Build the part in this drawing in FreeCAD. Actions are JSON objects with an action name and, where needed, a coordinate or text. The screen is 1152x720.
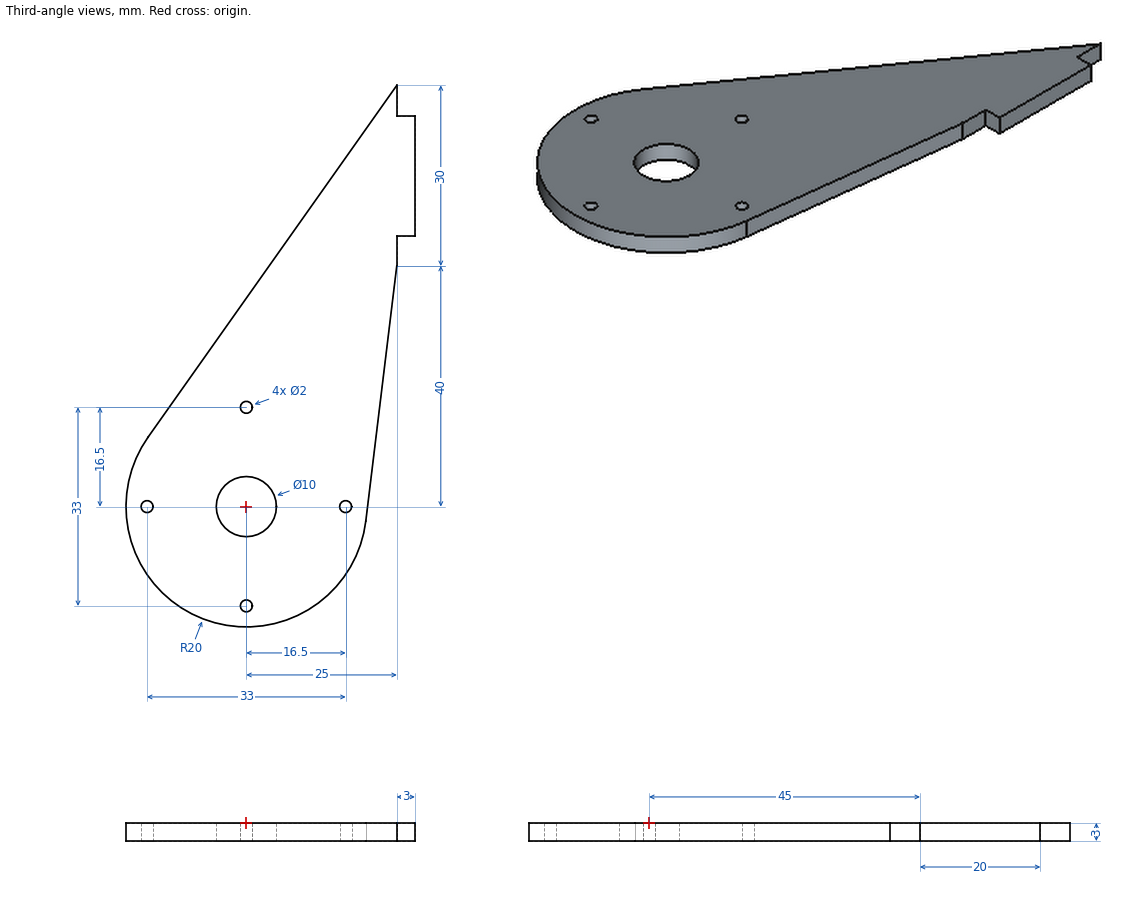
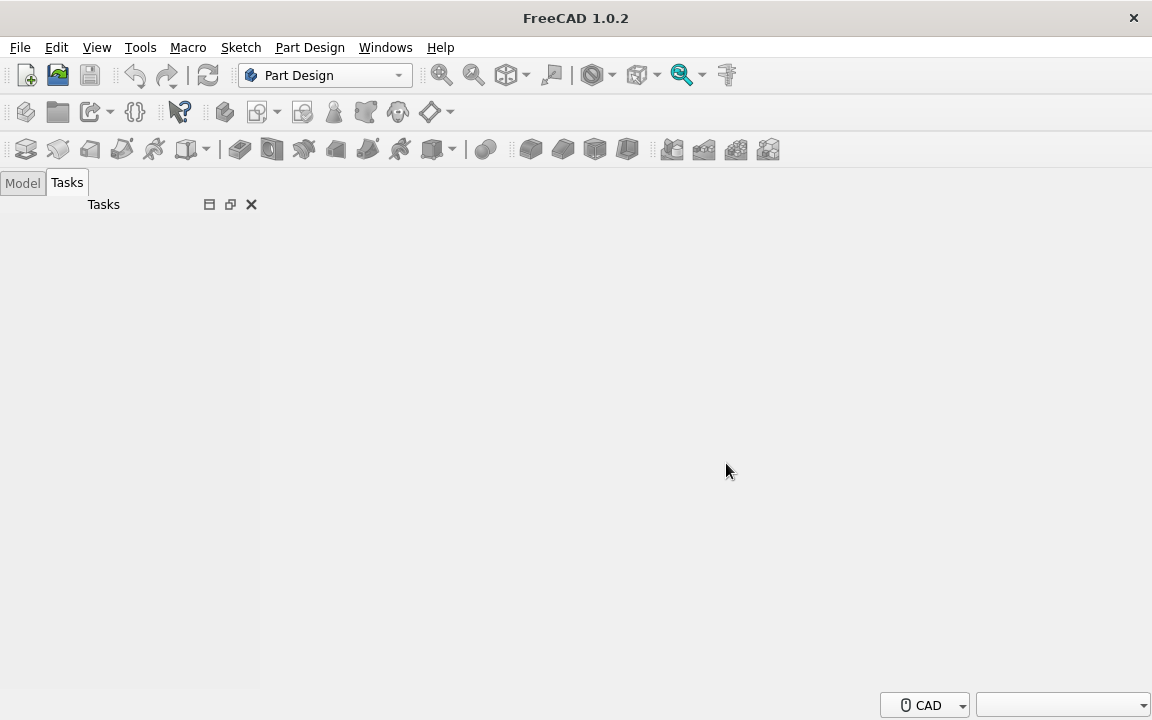
{"action": "left_click", "coordinate": [26, 76]}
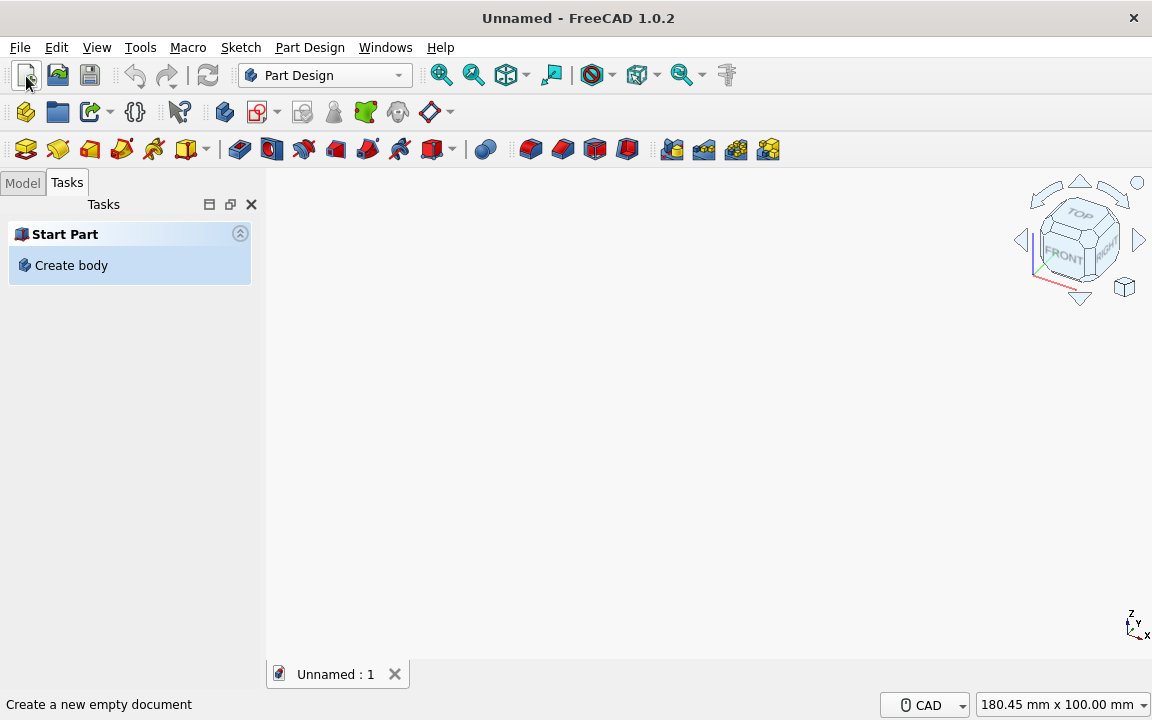
{"action": "left_click", "coordinate": [258, 112]}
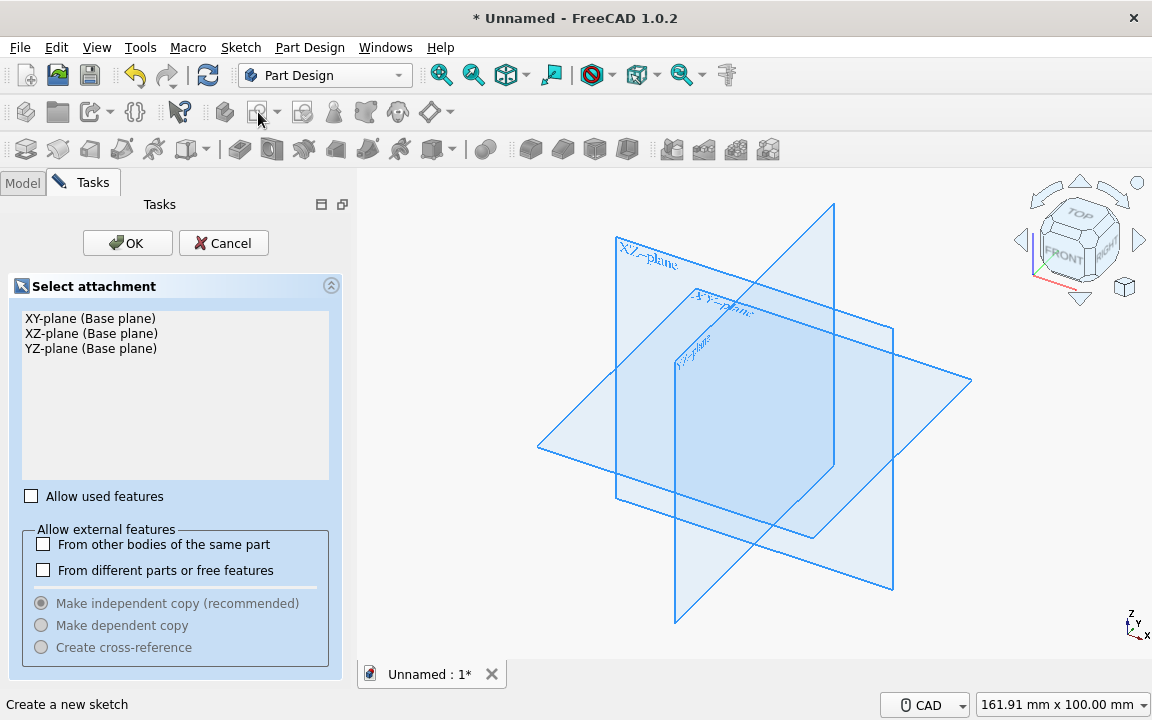
{"action": "left_click", "coordinate": [82, 318]}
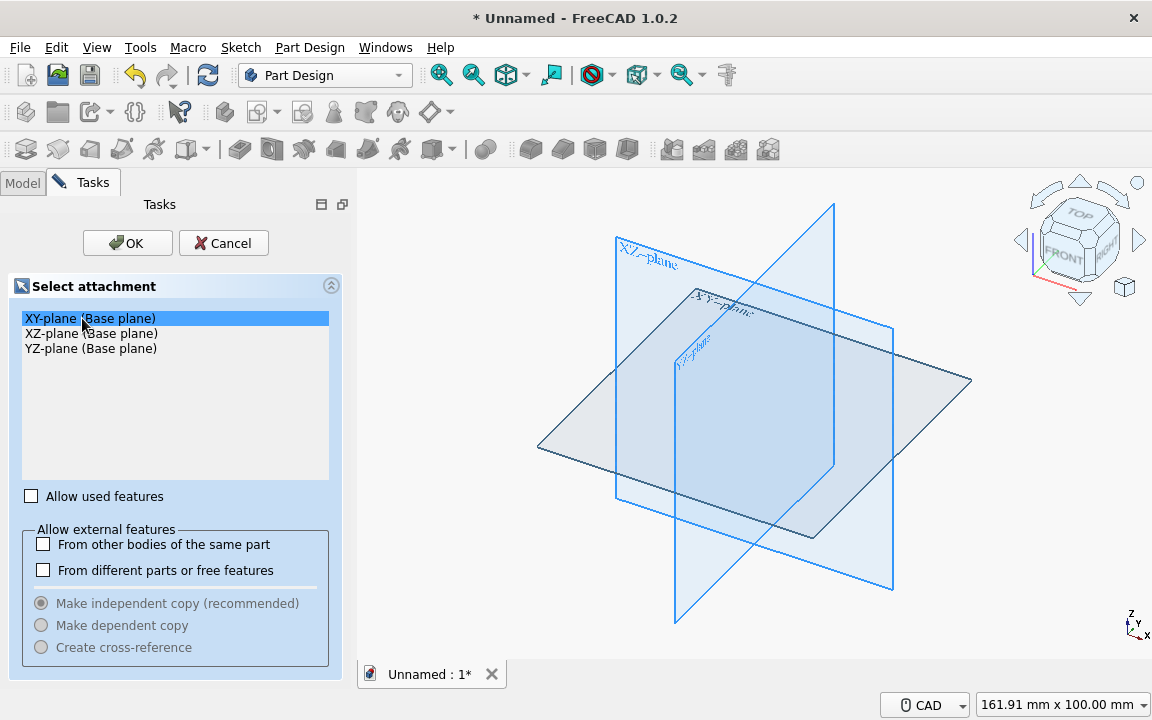
{"action": "left_click", "coordinate": [128, 243]}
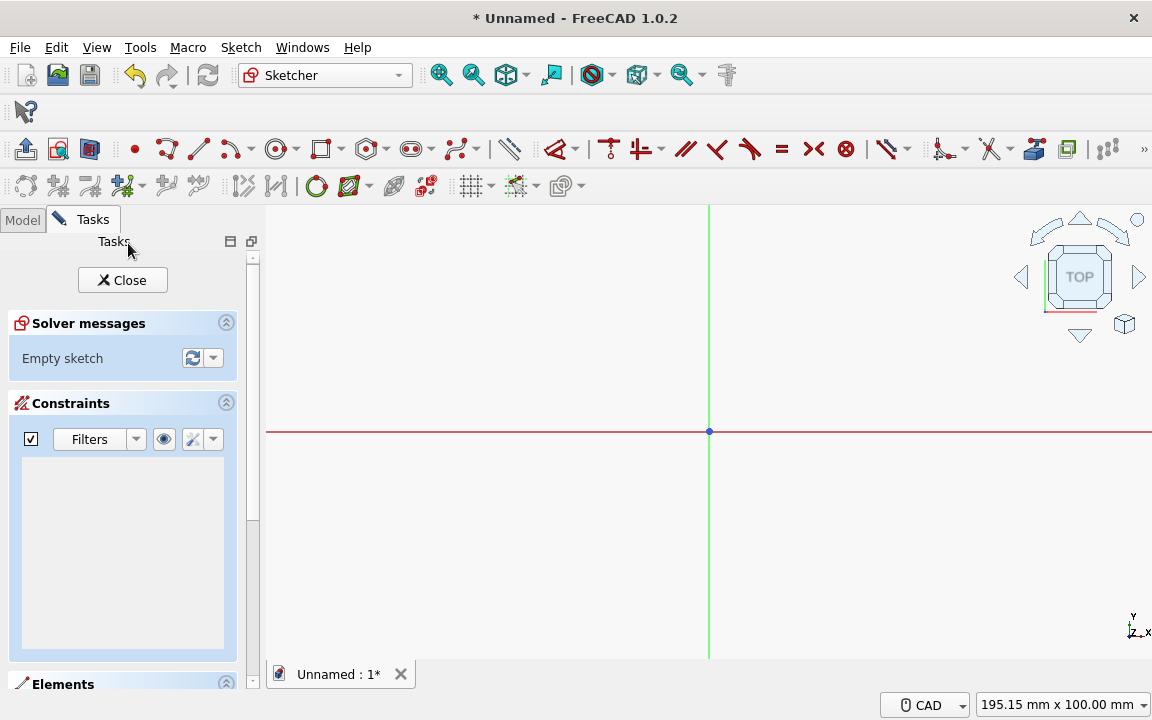
{"action": "scroll", "coordinate": [461, 631], "scroll_direction": "down", "scroll_amount": 2}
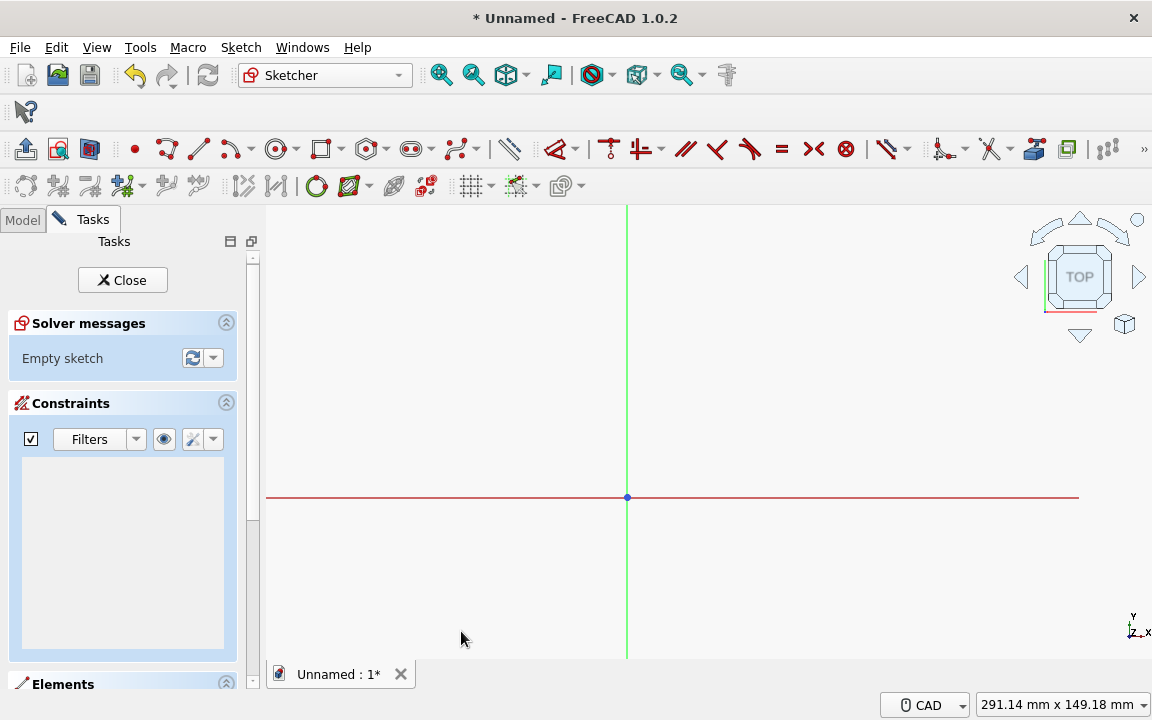
{"action": "left_click", "coordinate": [168, 150]}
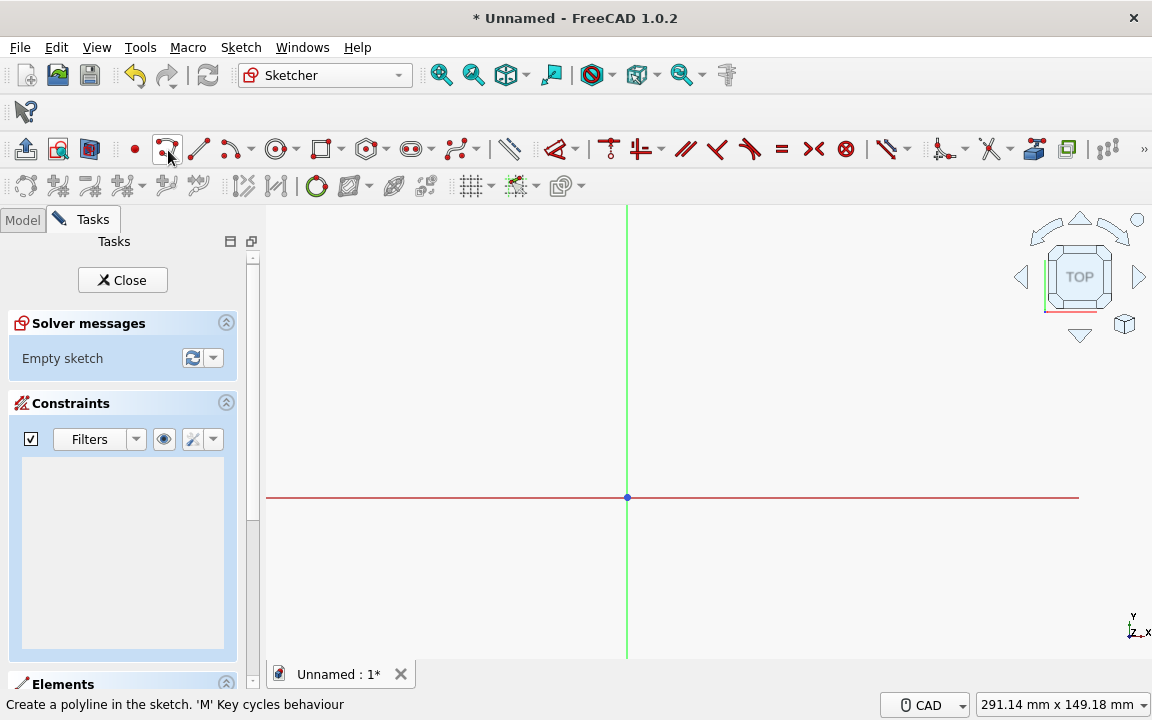
{"action": "scroll", "coordinate": [688, 505], "scroll_direction": "up", "scroll_amount": 4}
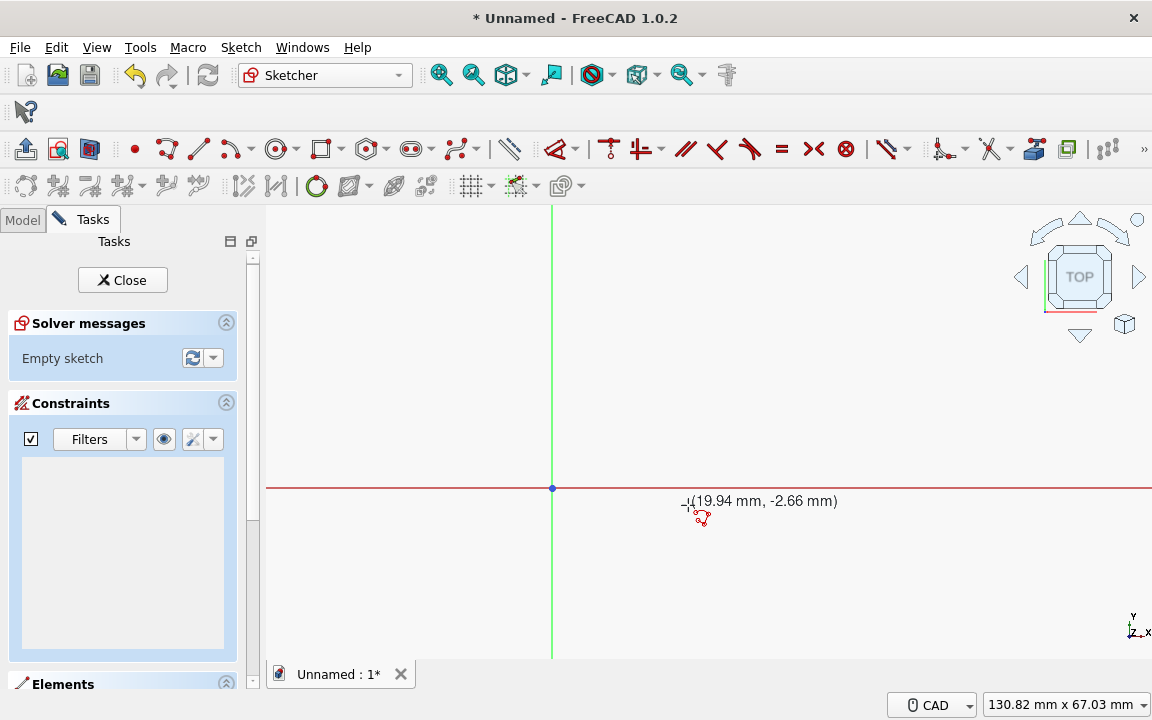
{"action": "left_click", "coordinate": [687, 505]}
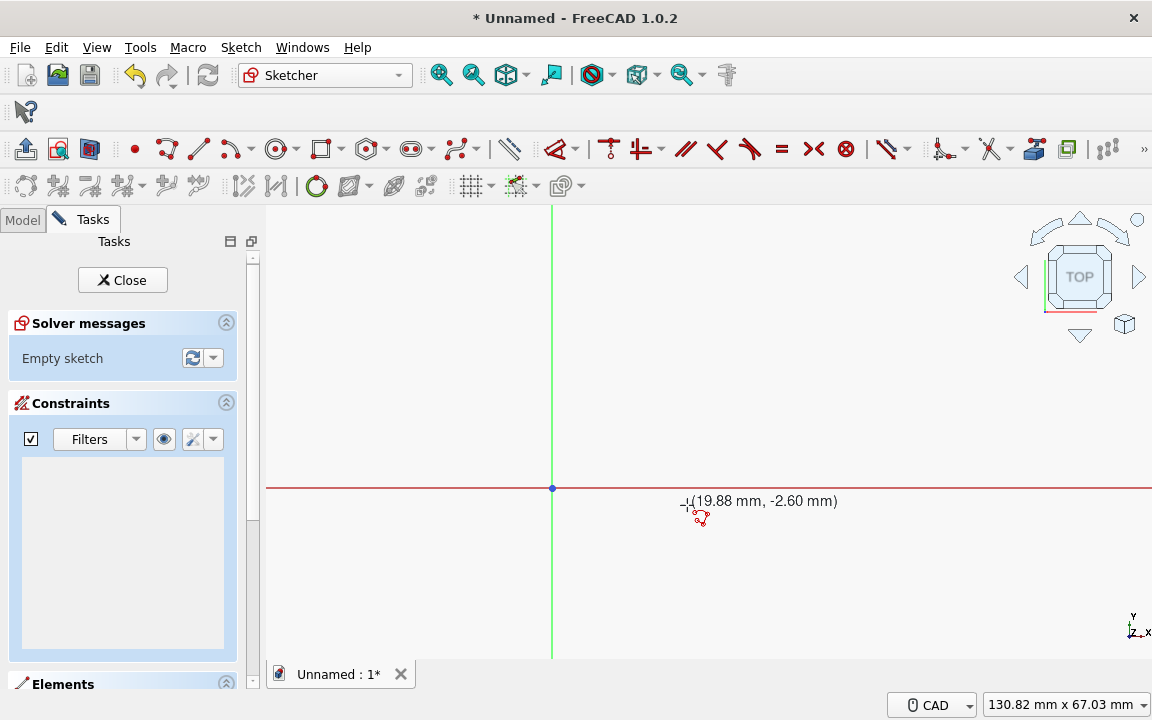
{"action": "scroll", "coordinate": [688, 528], "scroll_direction": "down", "scroll_amount": 4}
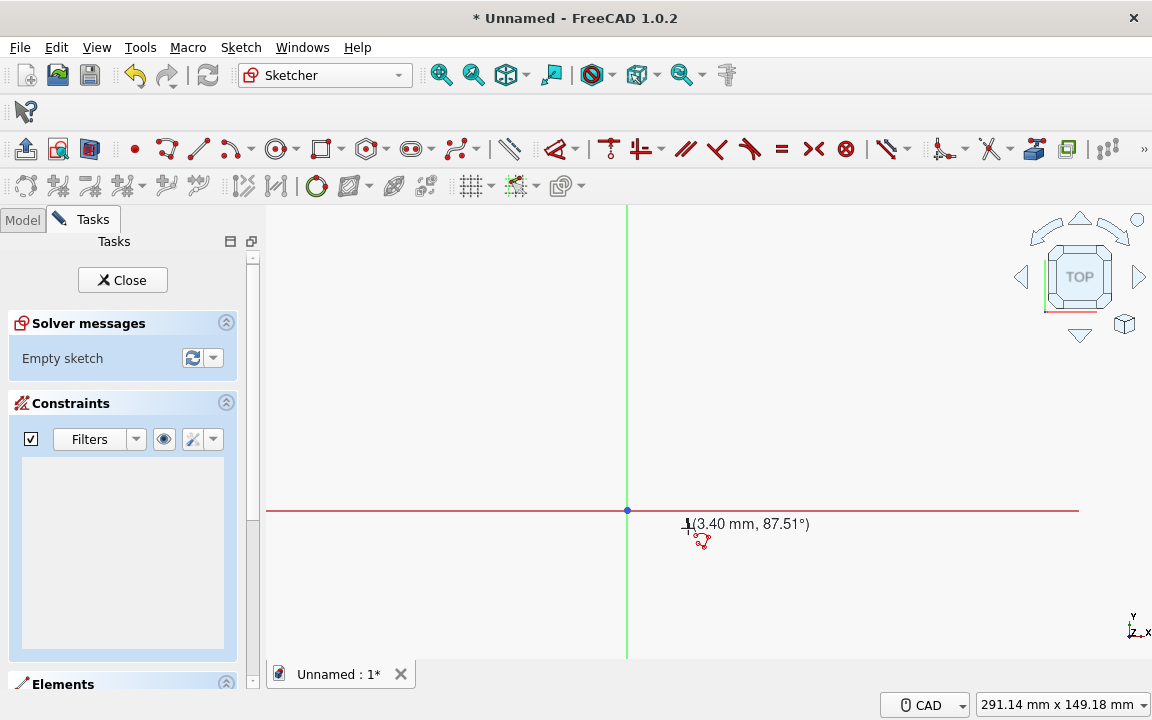
{"action": "left_click", "coordinate": [703, 389]}
{"action": "left_click", "coordinate": [703, 298]}
{"action": "left_click", "coordinate": [578, 475]}
{"action": "right_click", "coordinate": [578, 475]}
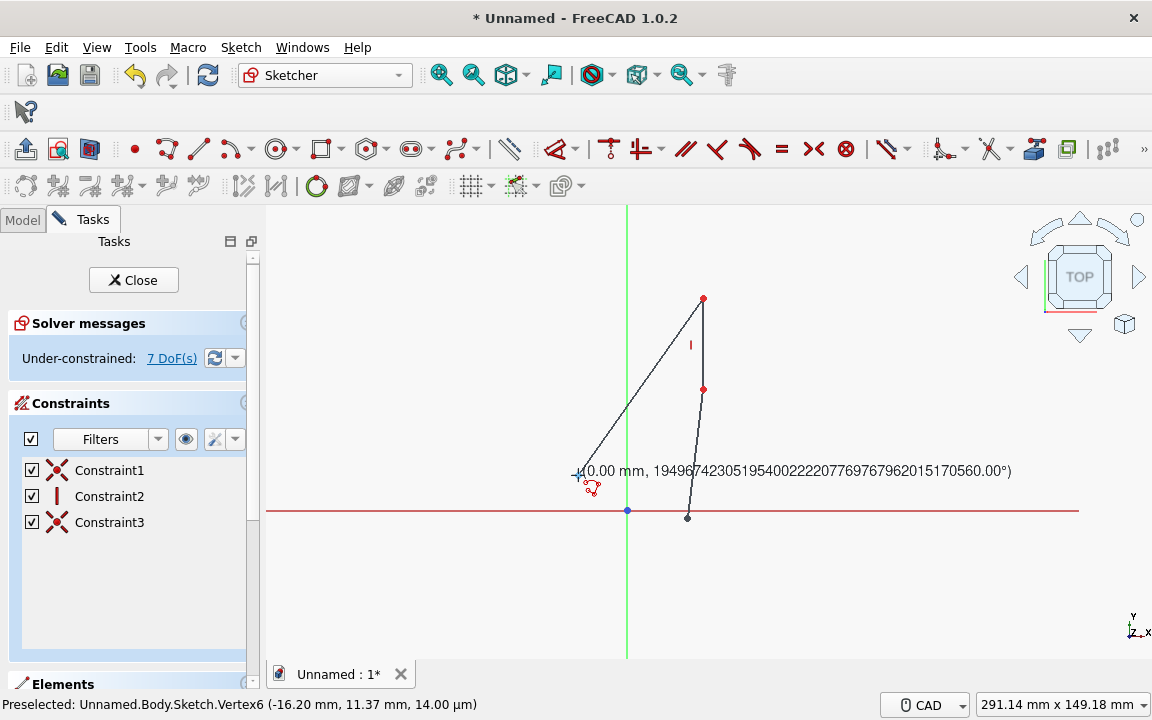
{"action": "left_click", "coordinate": [254, 150]}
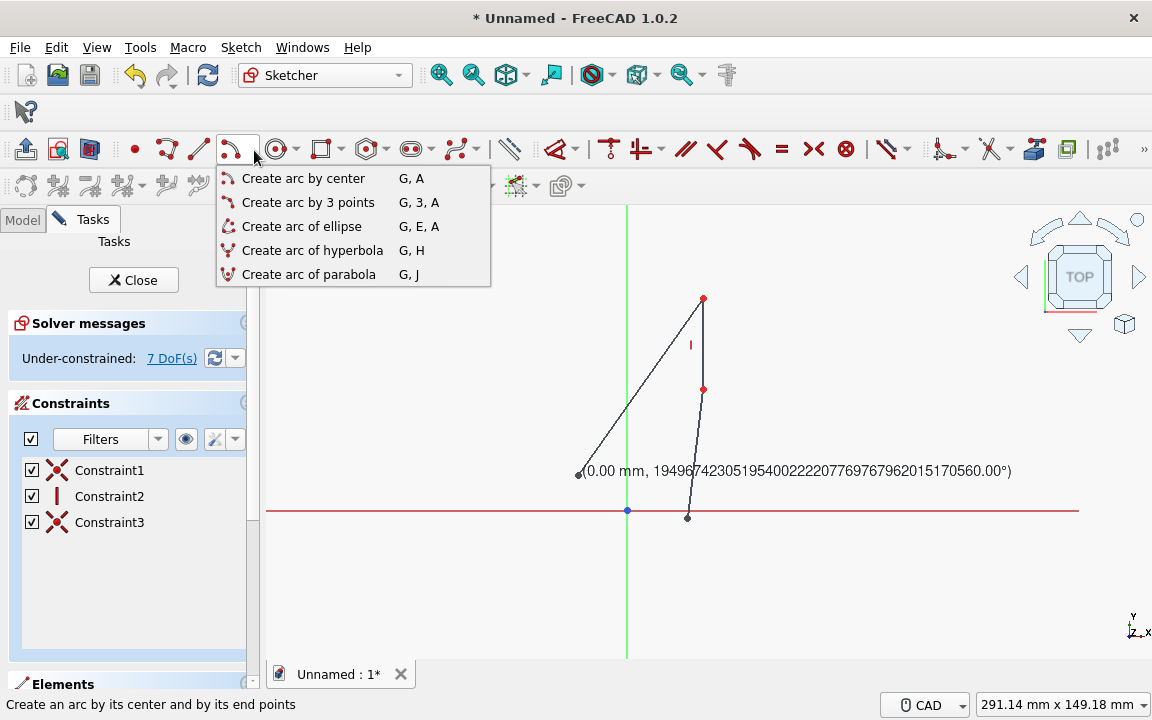
{"action": "left_click", "coordinate": [354, 202]}